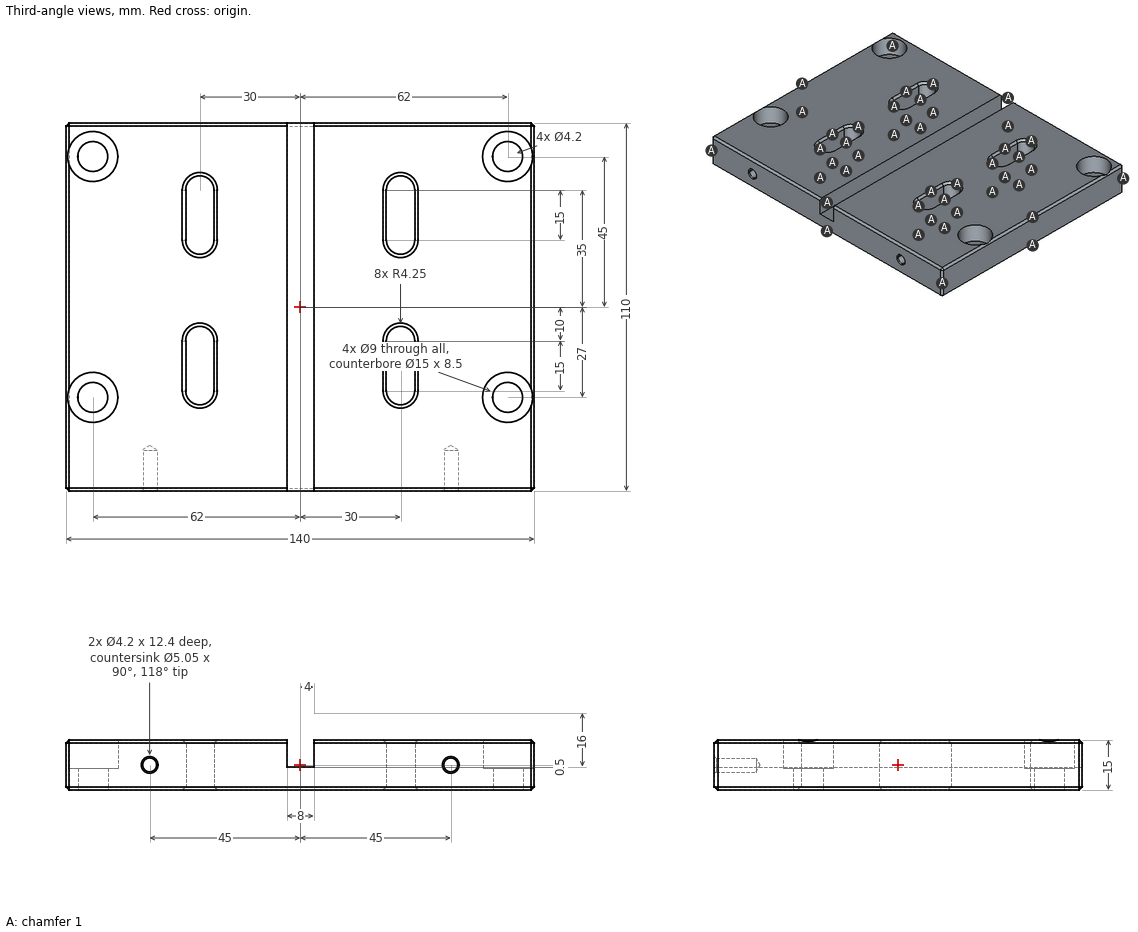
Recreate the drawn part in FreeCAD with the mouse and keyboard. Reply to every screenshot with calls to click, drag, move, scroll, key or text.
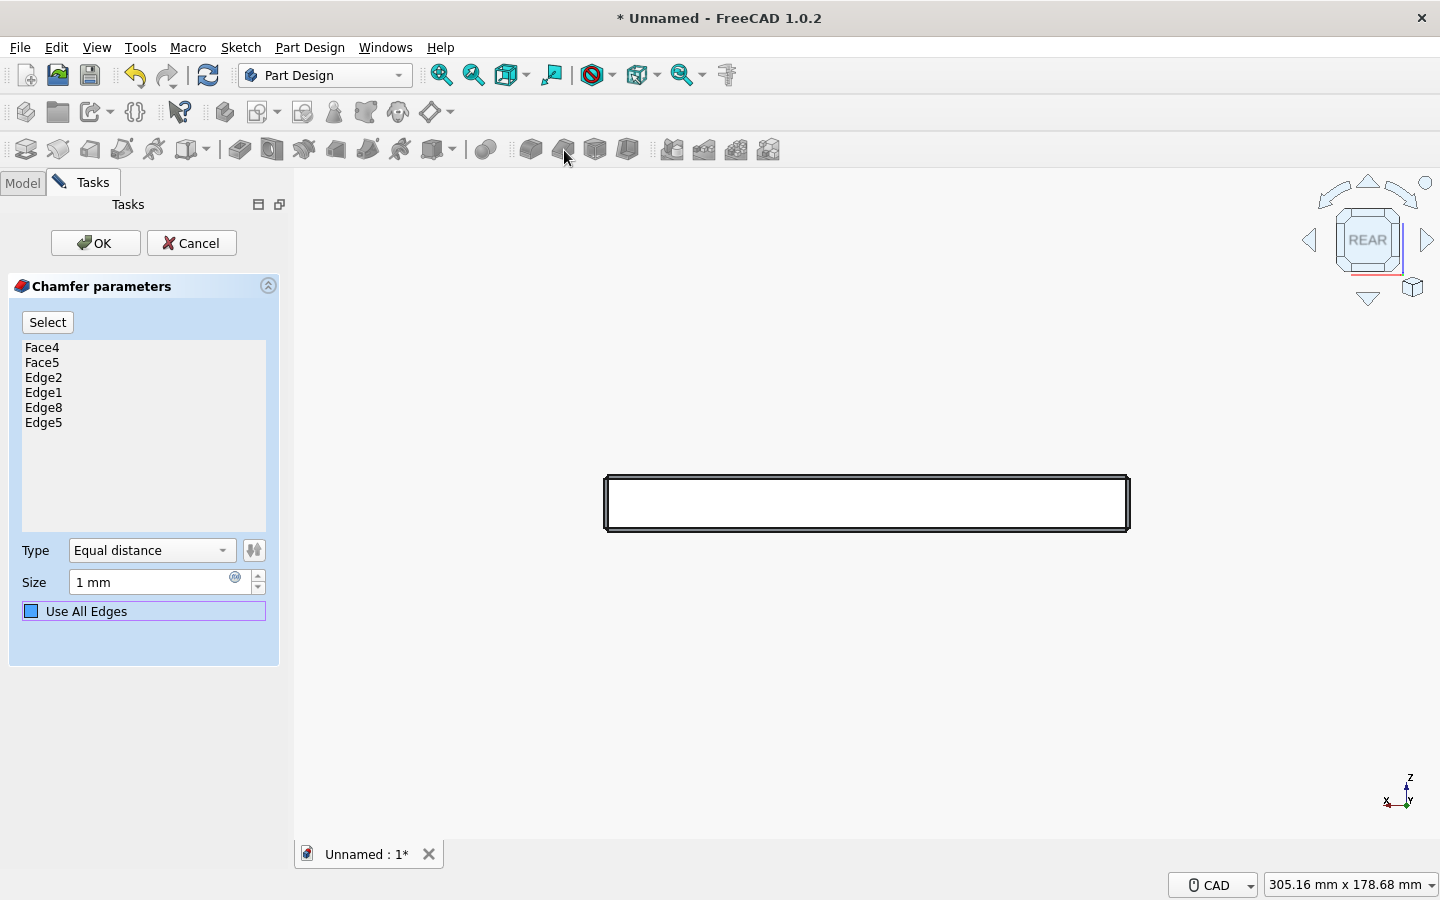
click(96, 243)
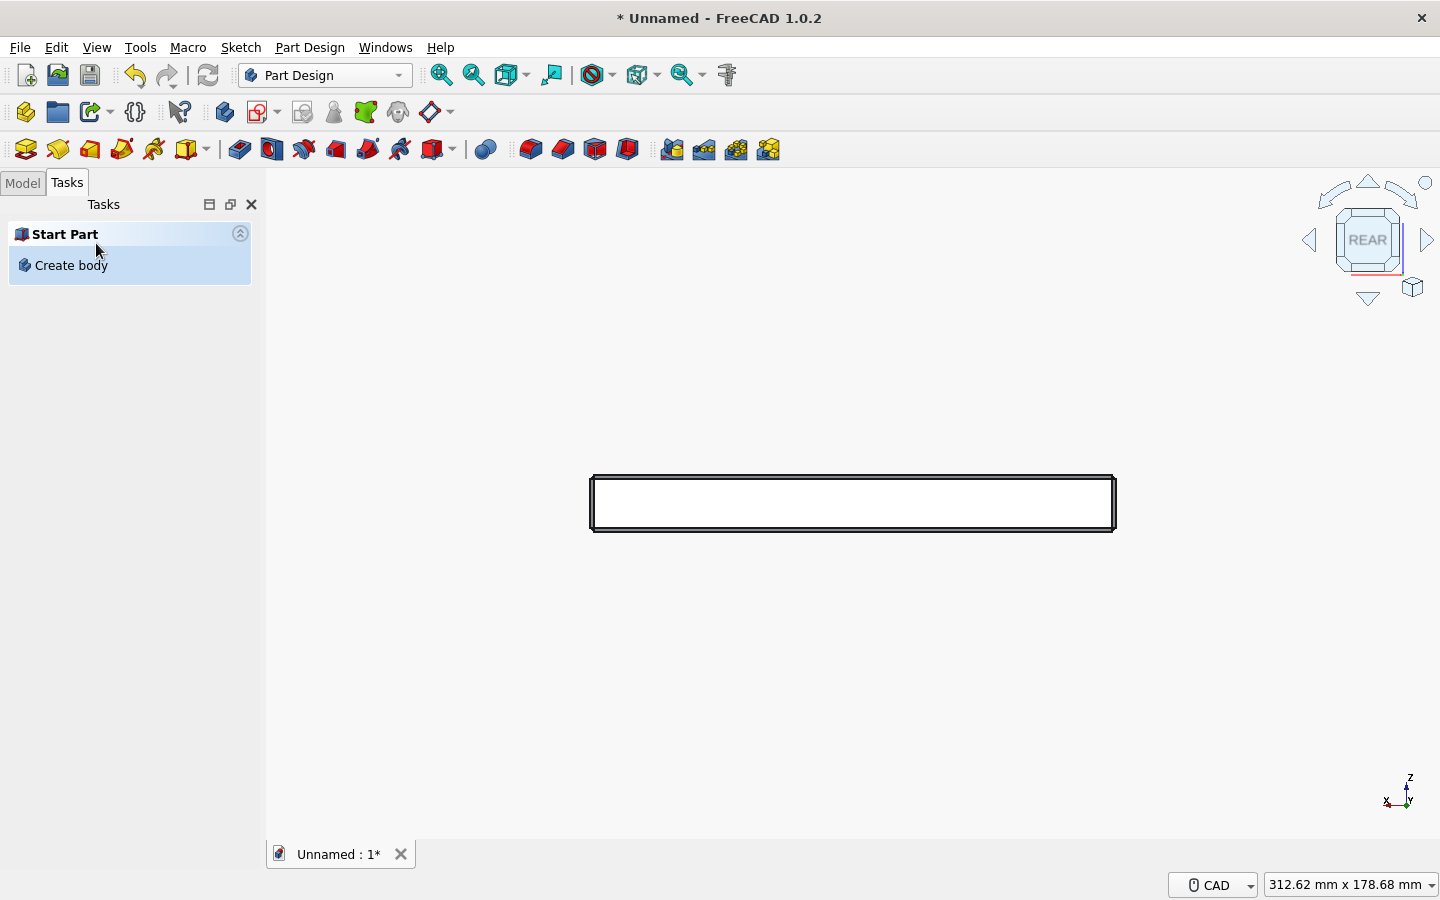
key(v)
key(f)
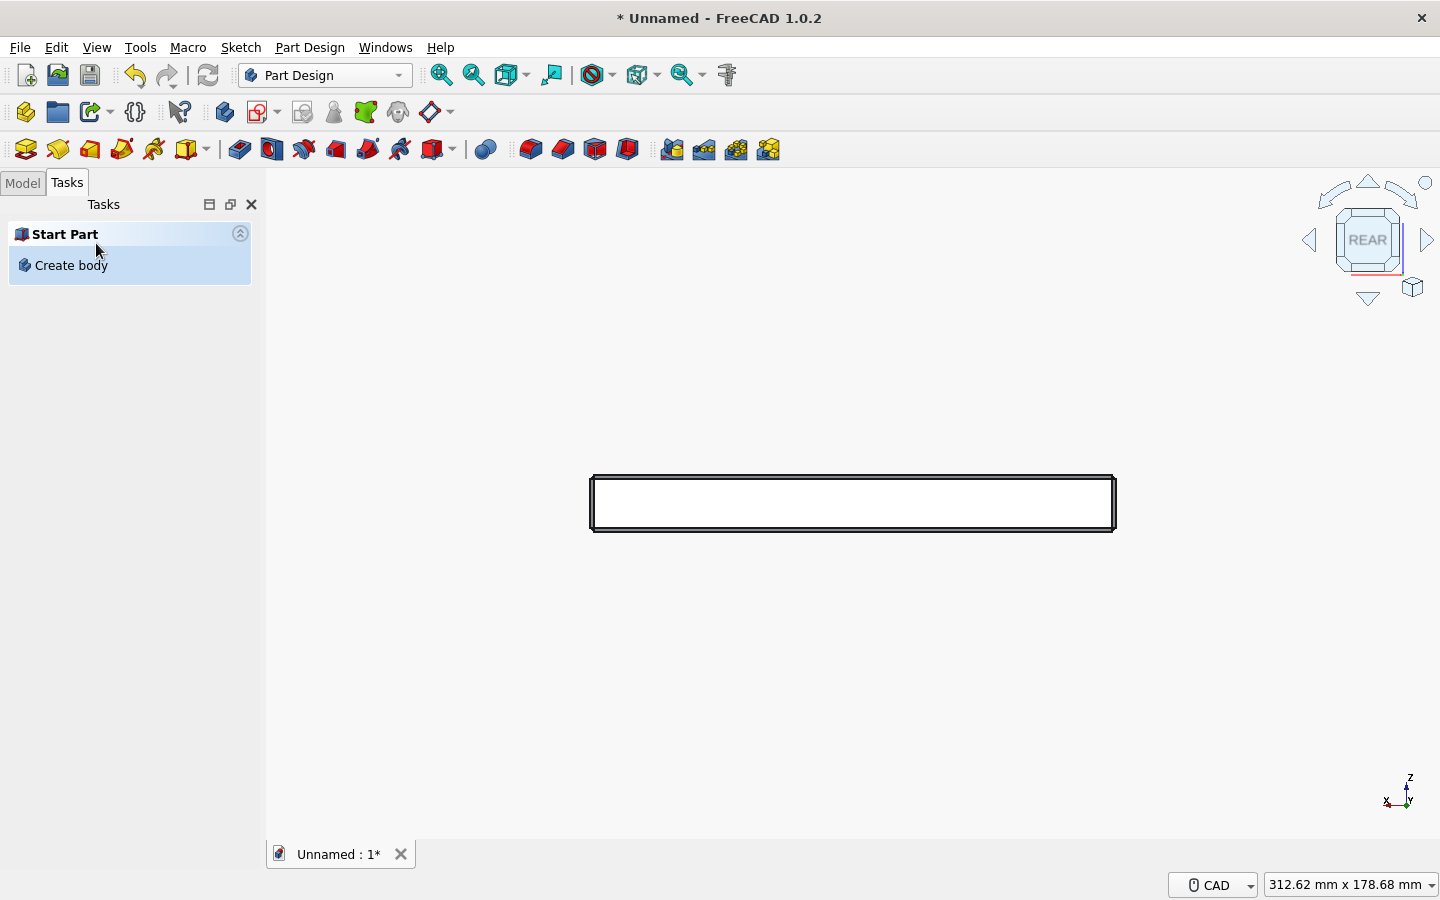
click(631, 503)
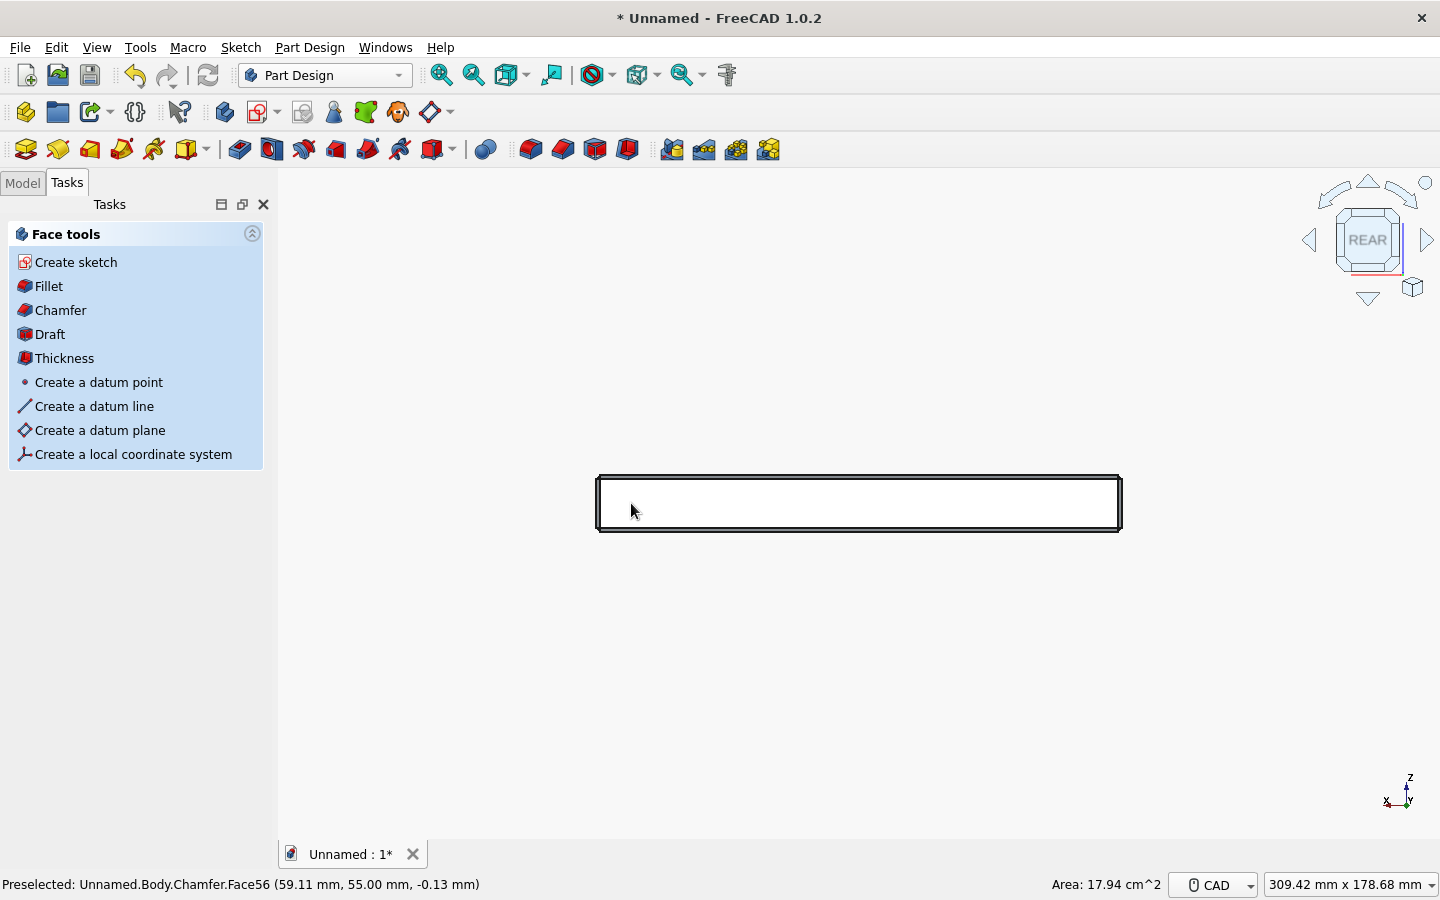
click(258, 112)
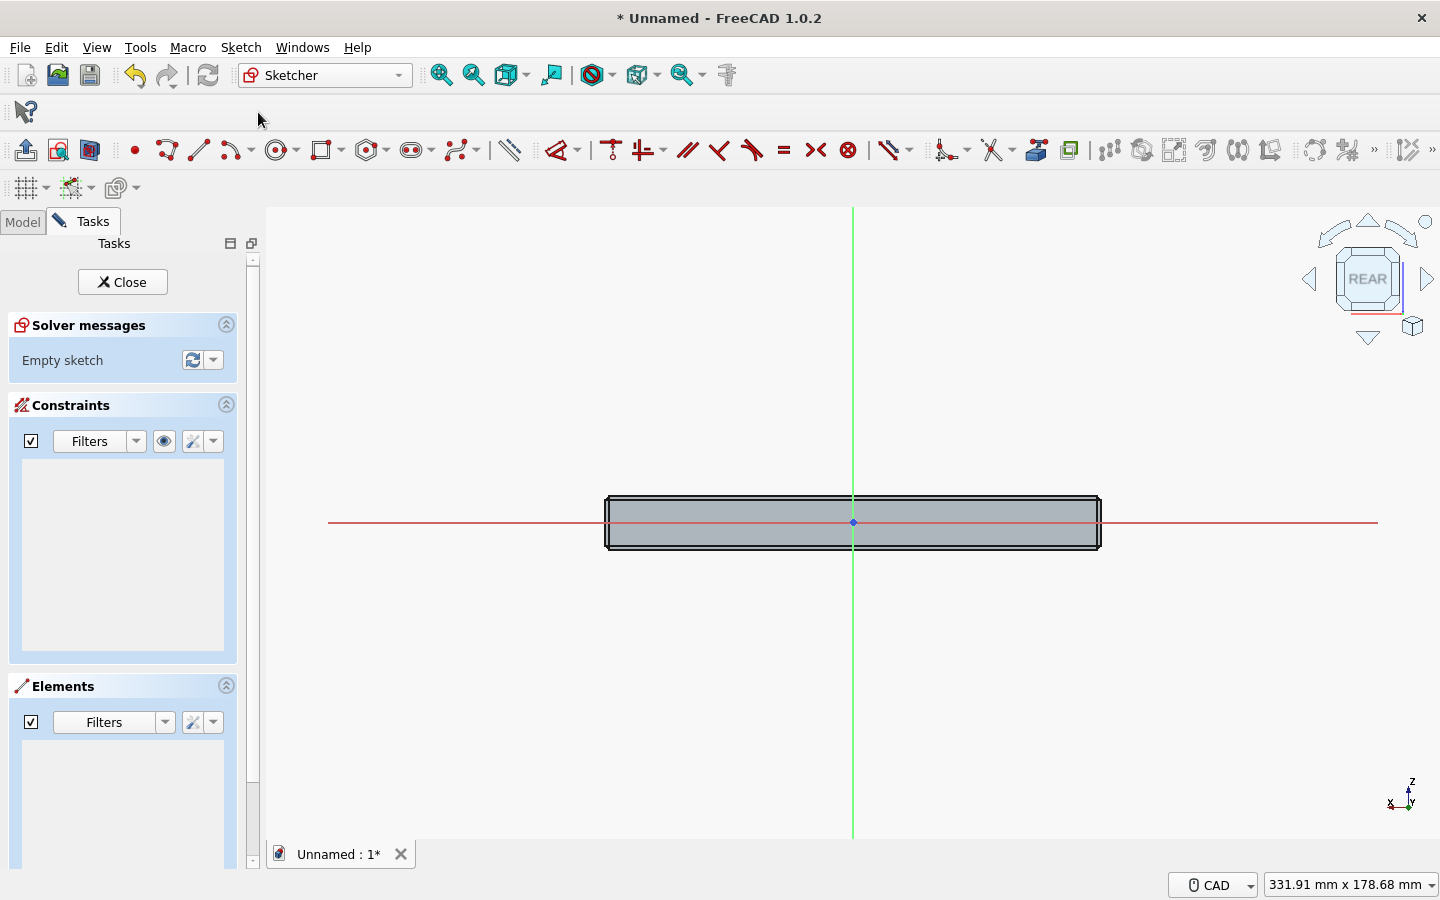
scroll(864, 492, up, 10)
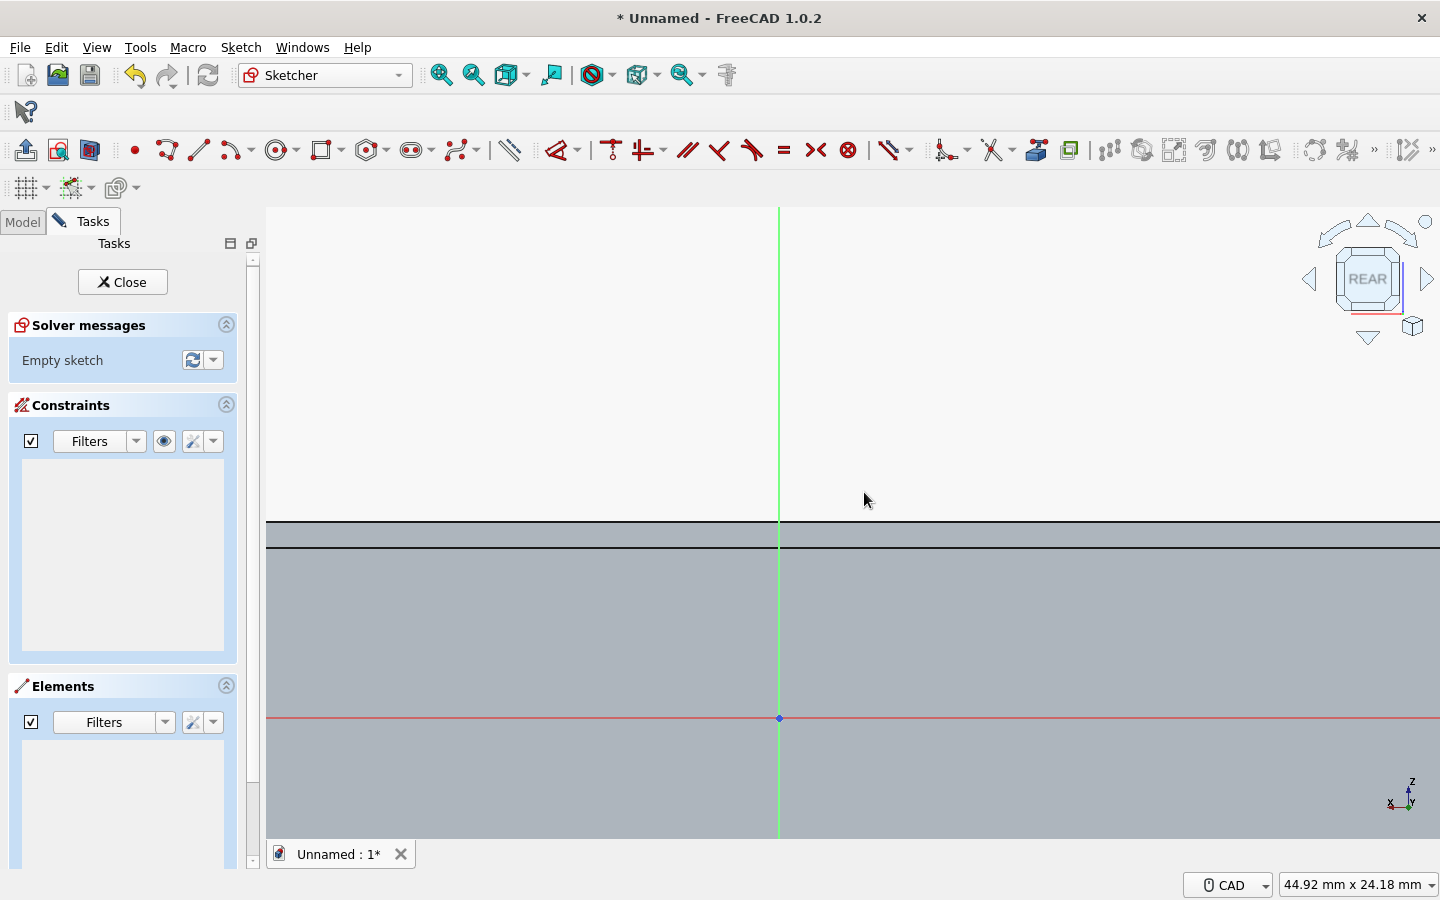
click(322, 150)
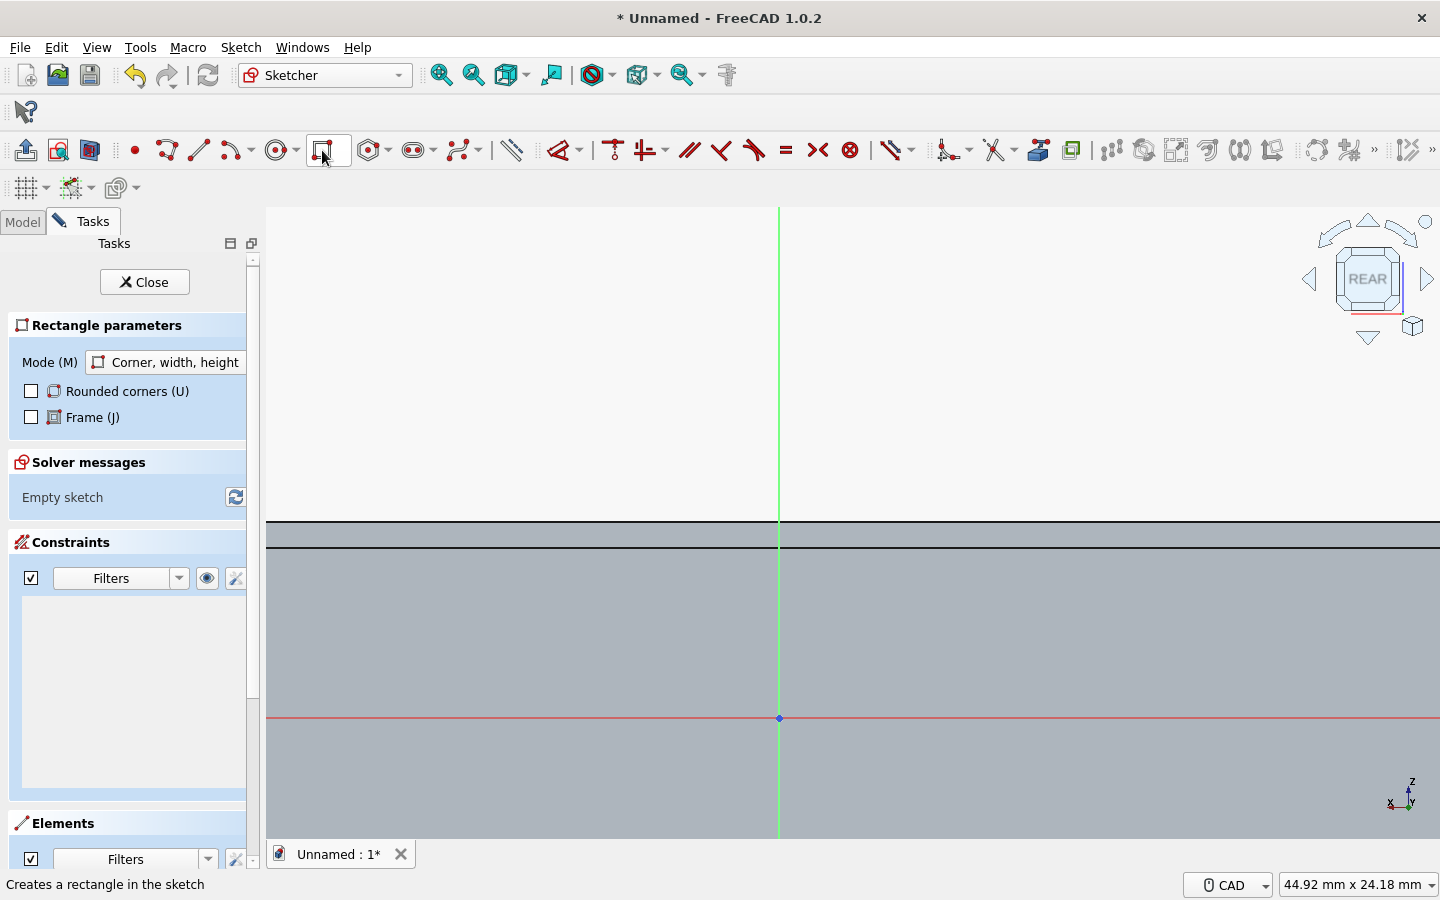
click(675, 313)
click(884, 731)
key(Escape)